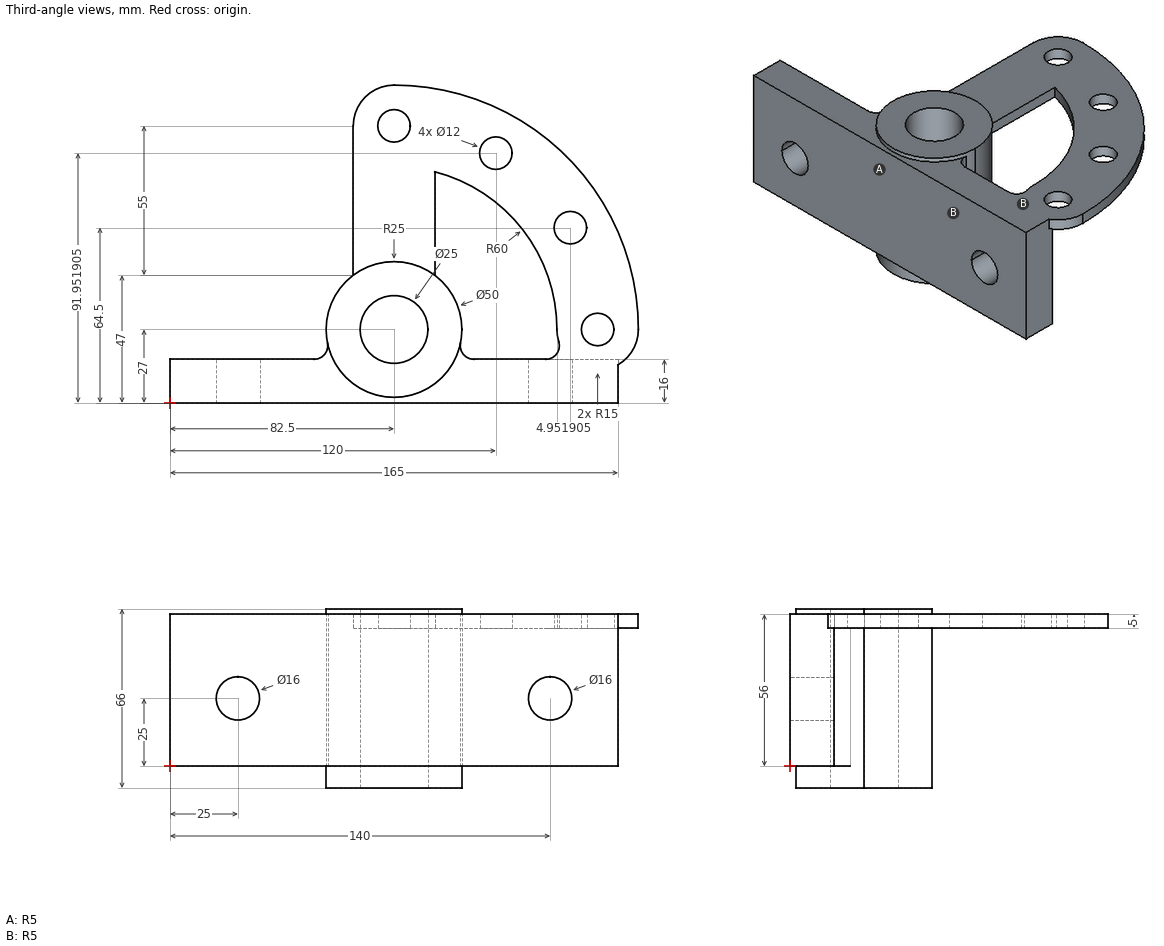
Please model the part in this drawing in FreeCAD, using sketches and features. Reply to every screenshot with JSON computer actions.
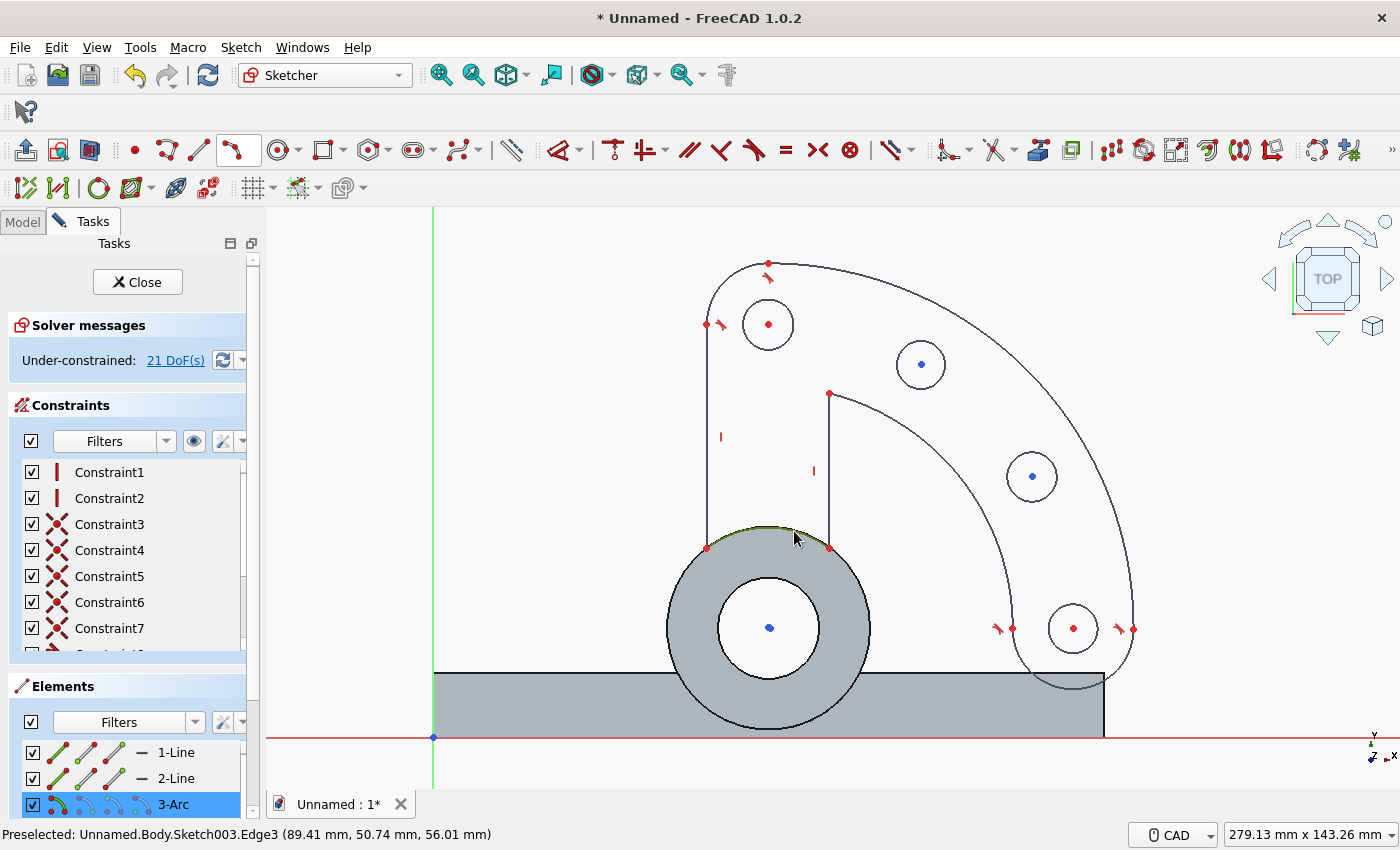
{"action": "left_click", "coordinate": [994, 535]}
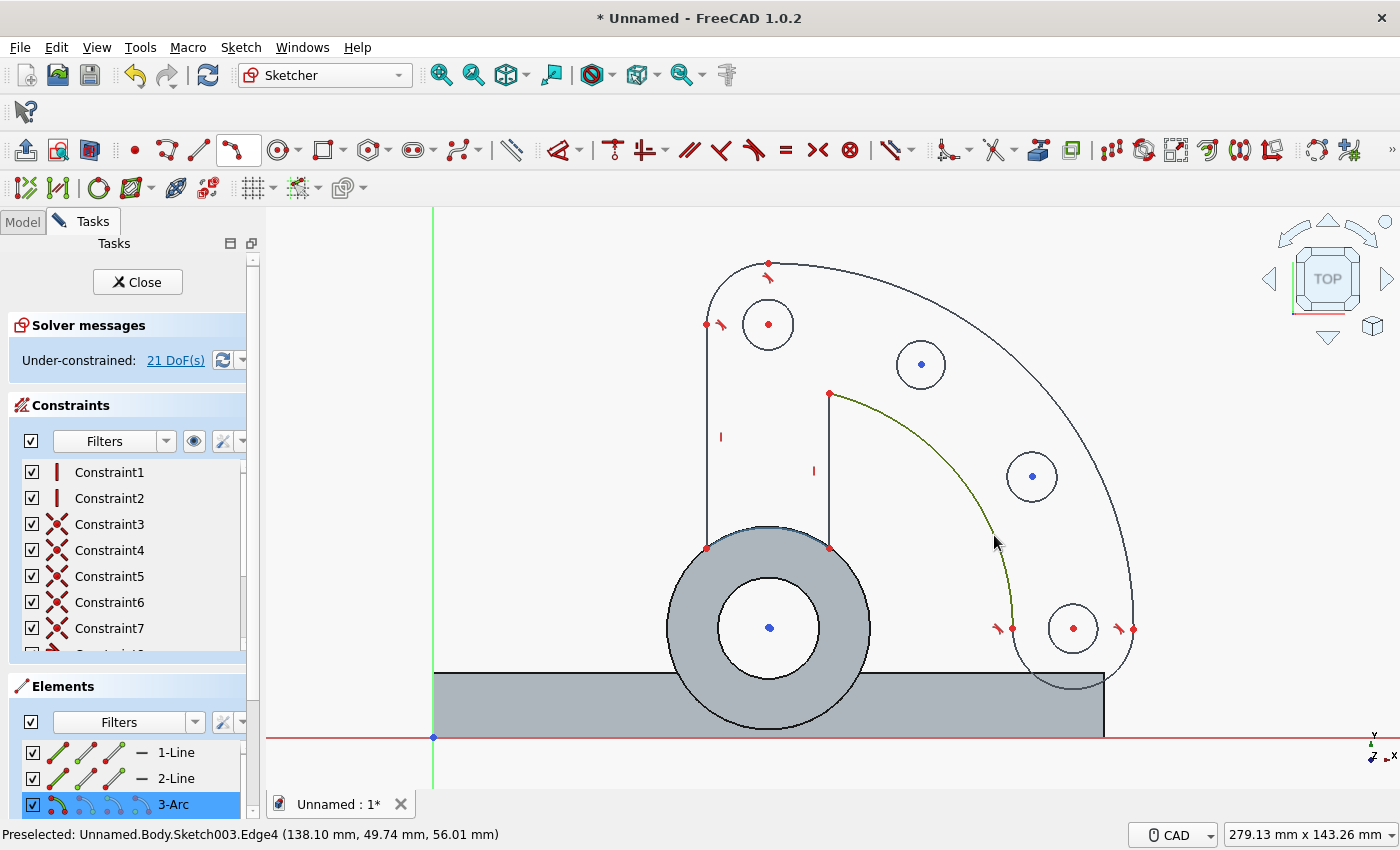
{"action": "left_click", "coordinate": [614, 150]}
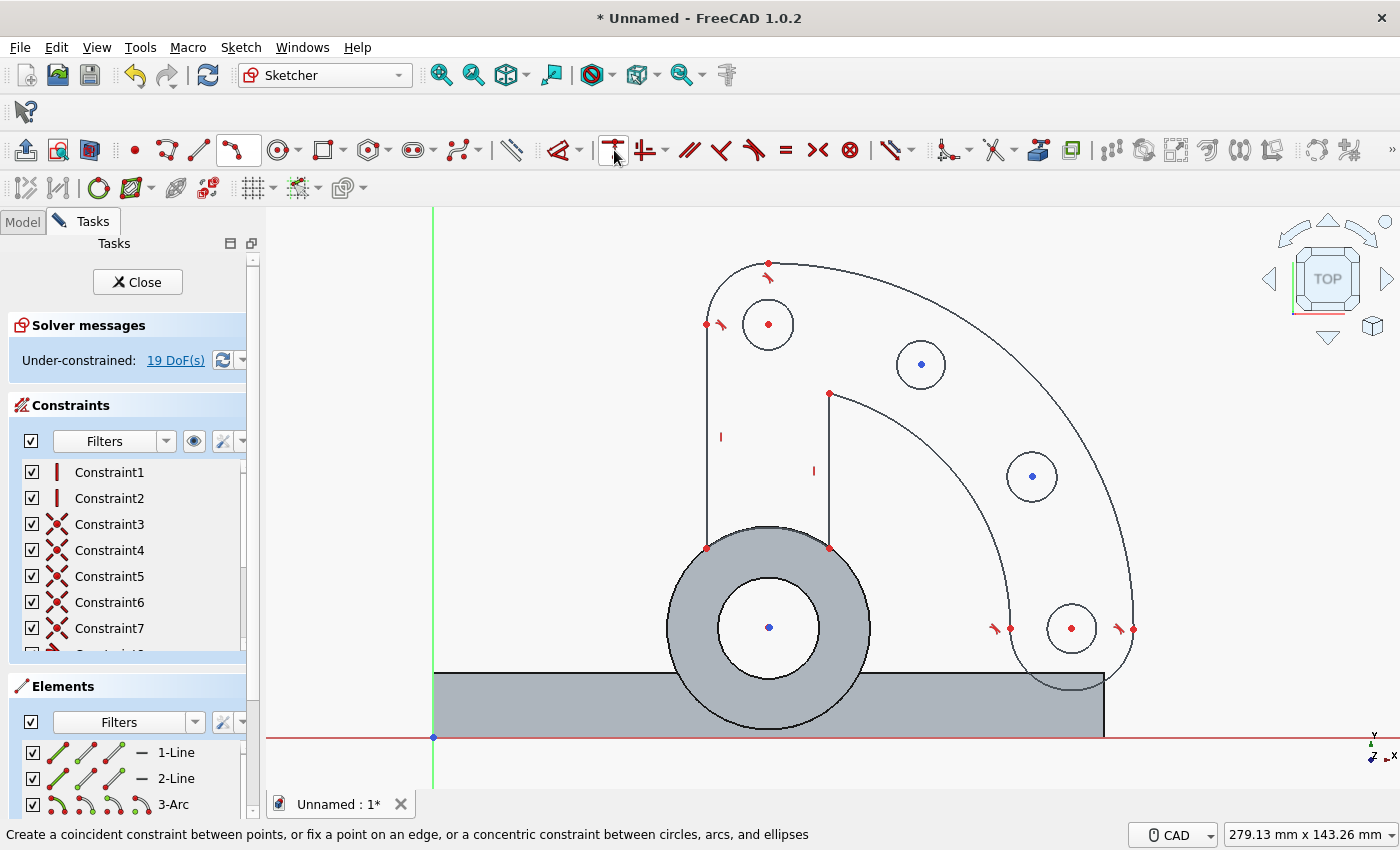
{"action": "left_click", "coordinate": [794, 531]}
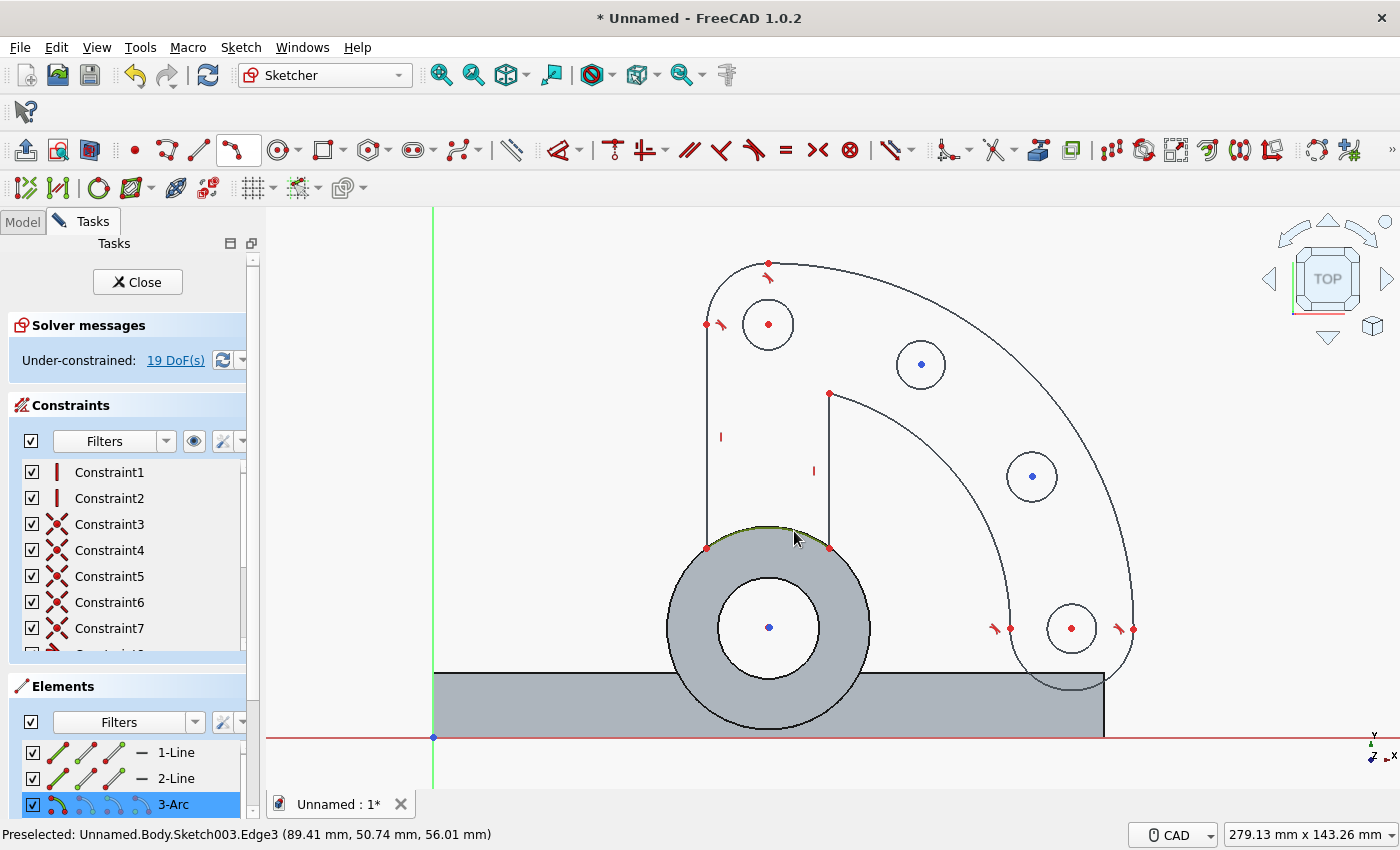
{"action": "left_click", "coordinate": [1094, 463]}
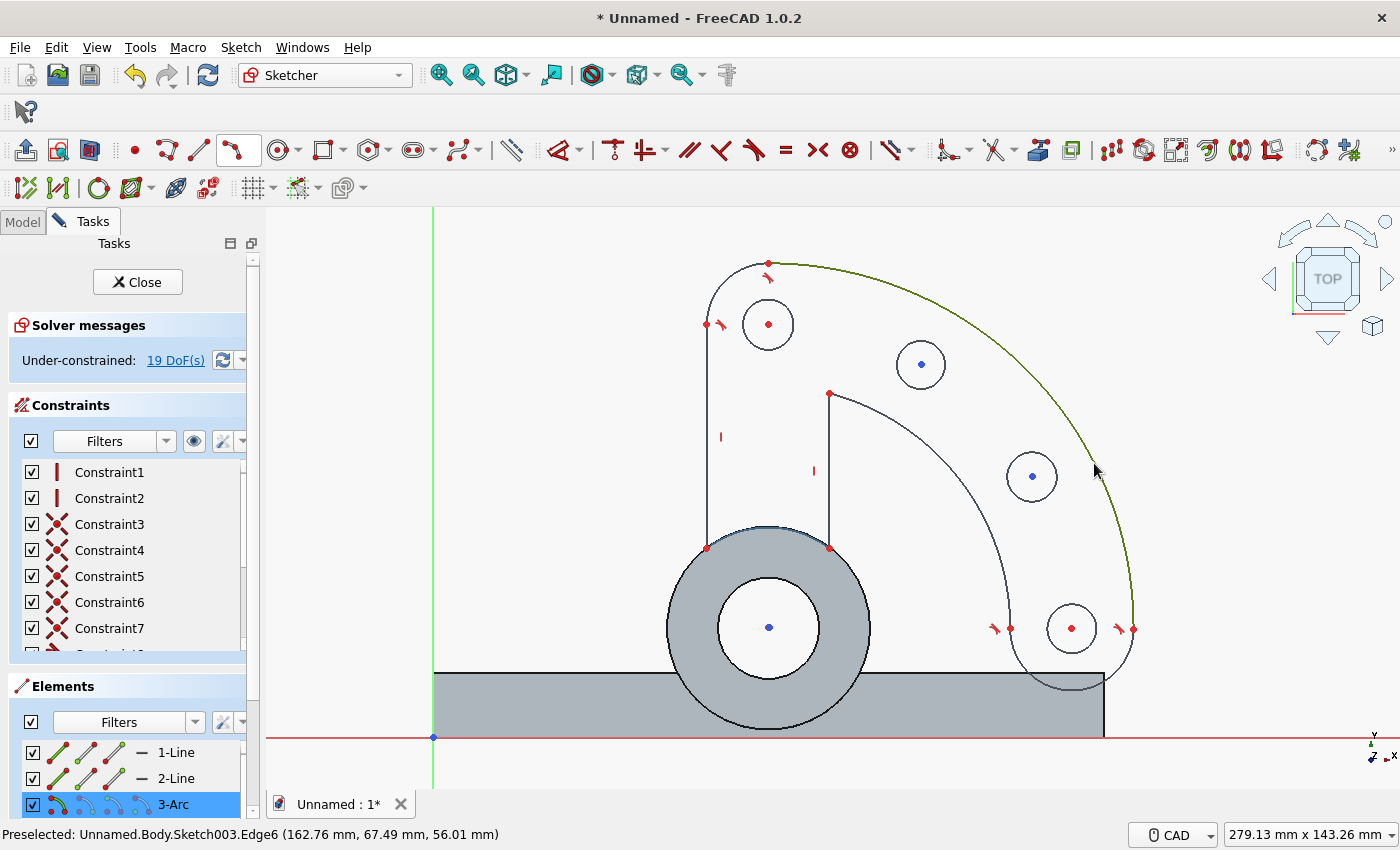
{"action": "left_click", "coordinate": [614, 150]}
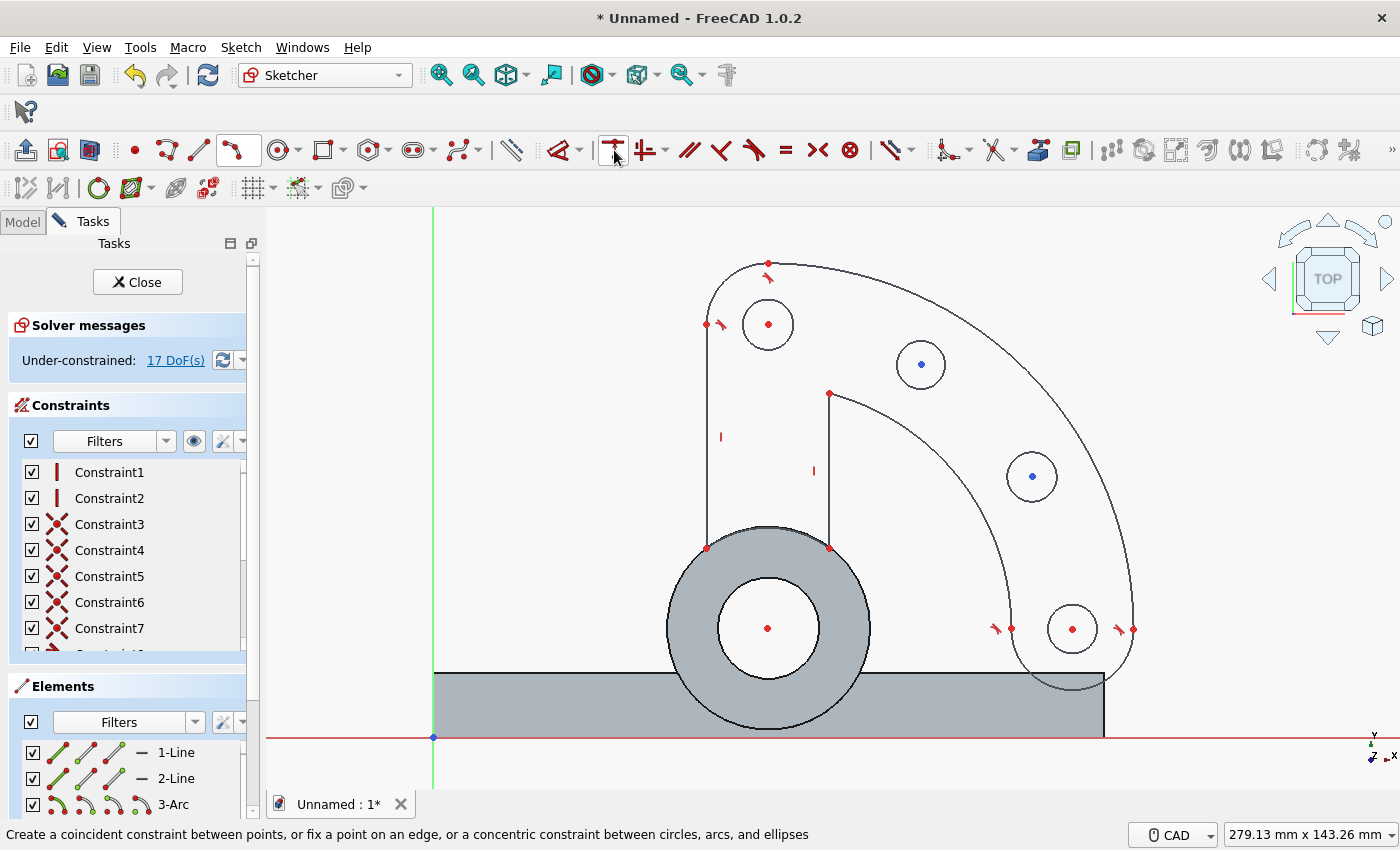
{"action": "left_click", "coordinate": [1037, 678]}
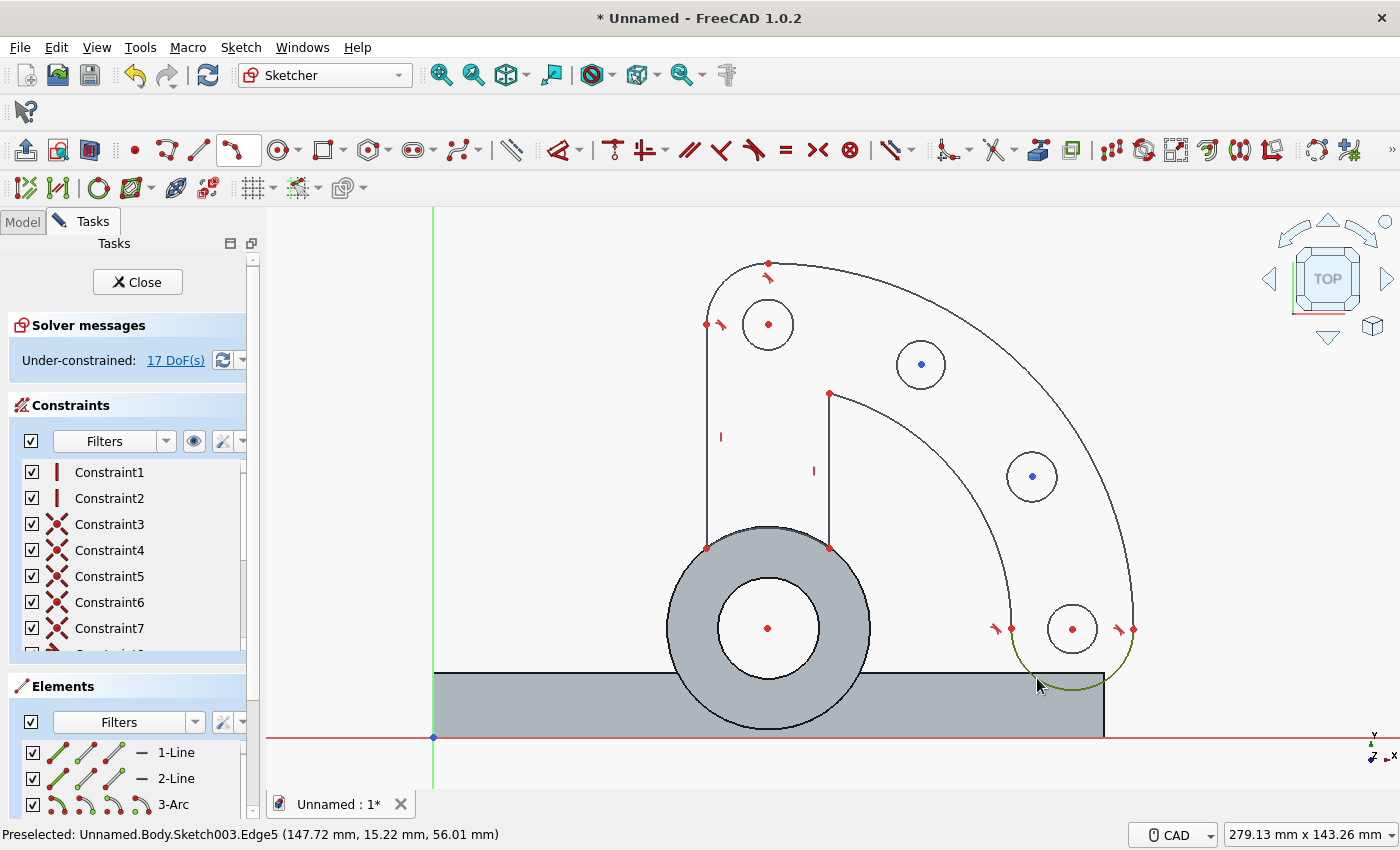
{"action": "left_click", "coordinate": [740, 270]}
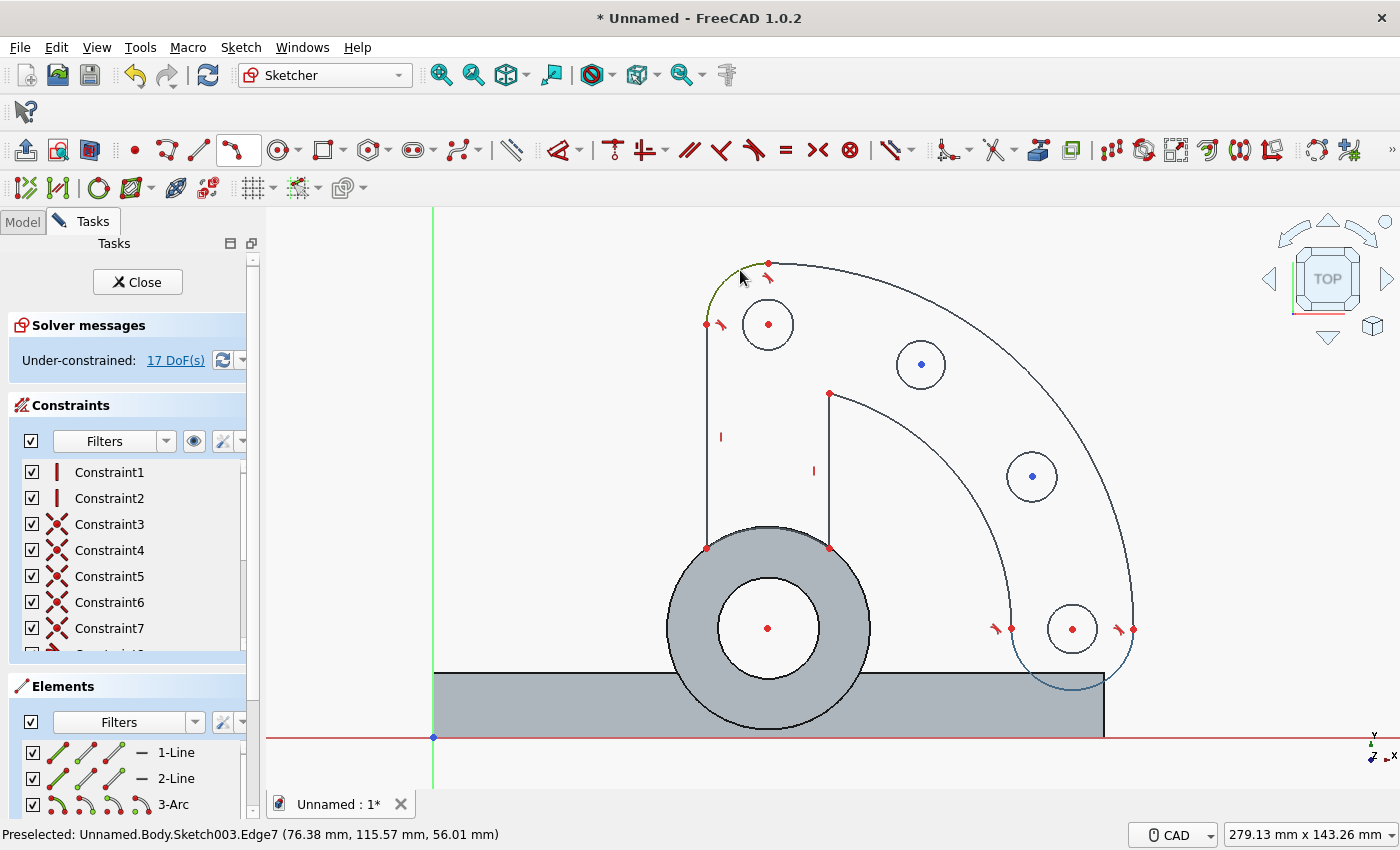
{"action": "left_click", "coordinate": [786, 150]}